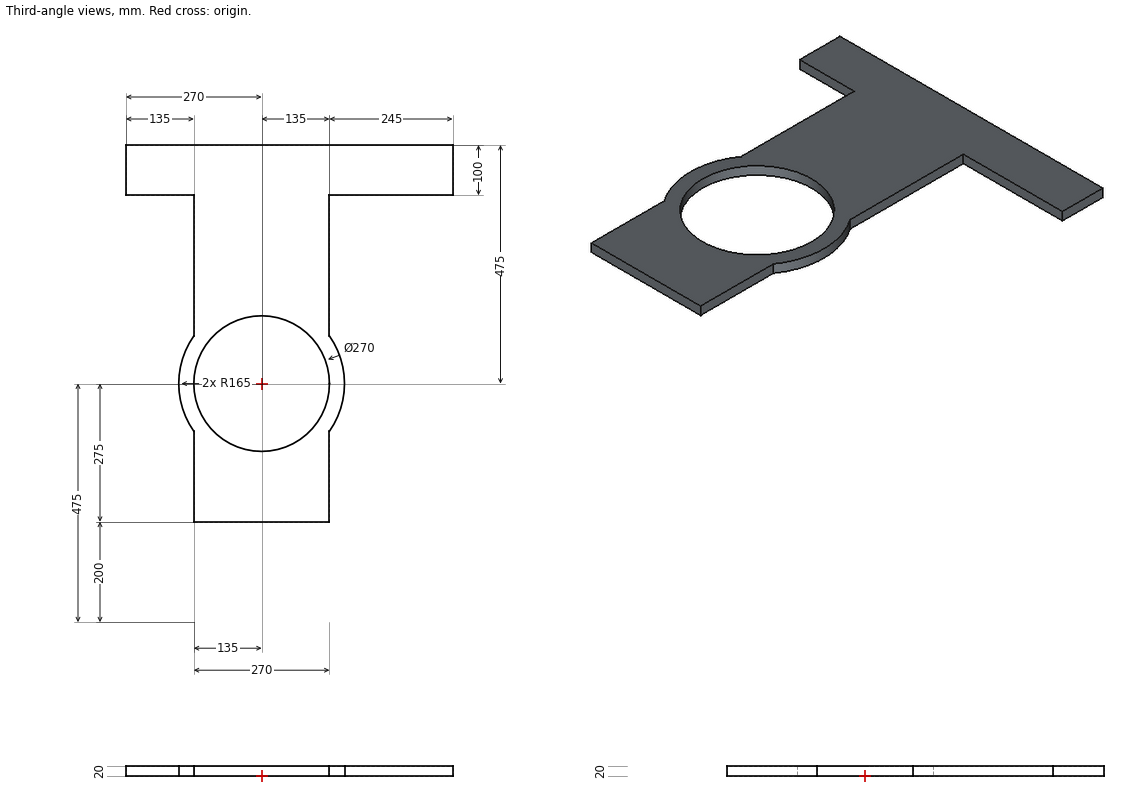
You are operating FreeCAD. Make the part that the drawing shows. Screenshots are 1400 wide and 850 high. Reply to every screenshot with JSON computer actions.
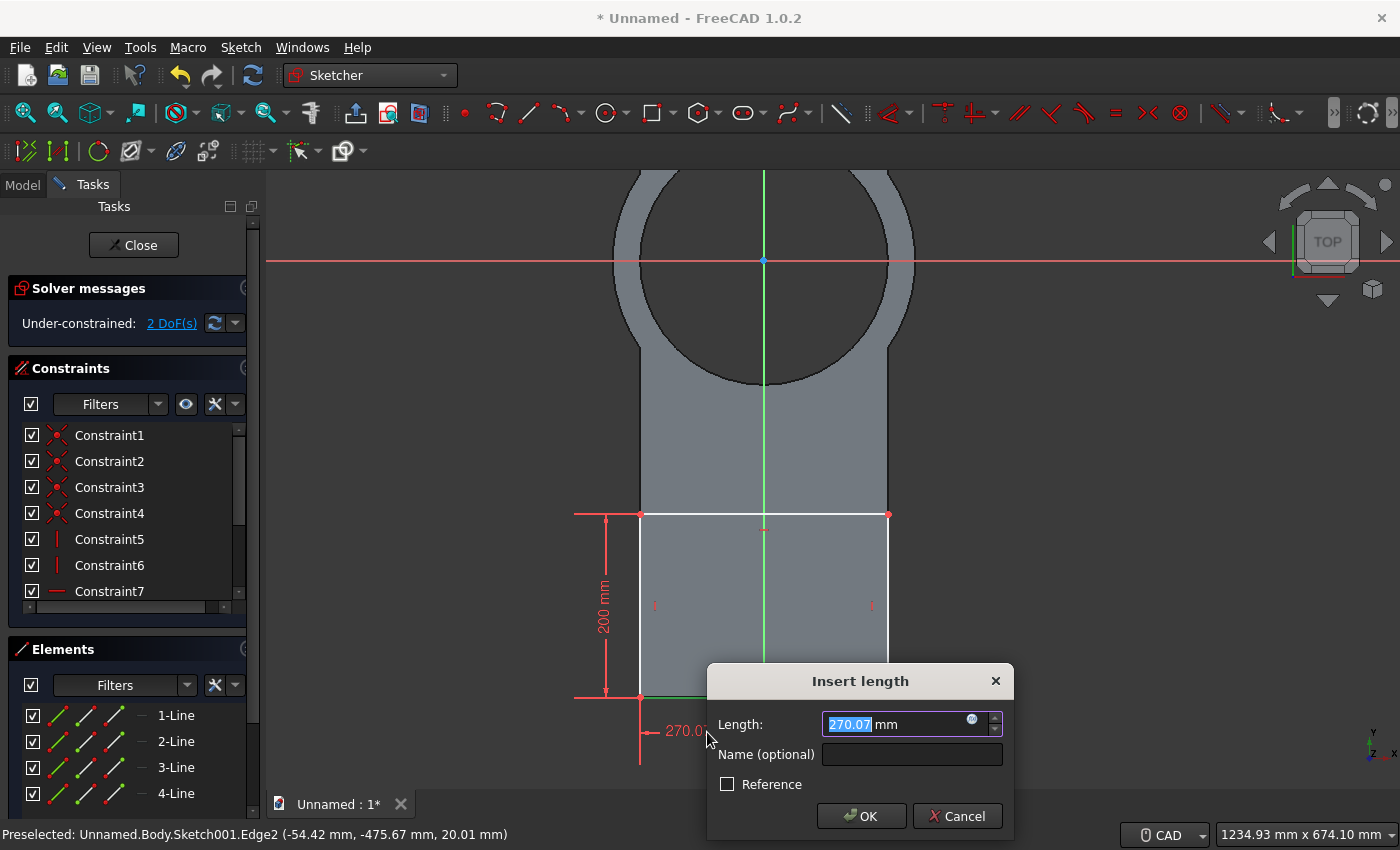
{"action": "type", "text": "270"}
{"action": "key", "text": "Return"}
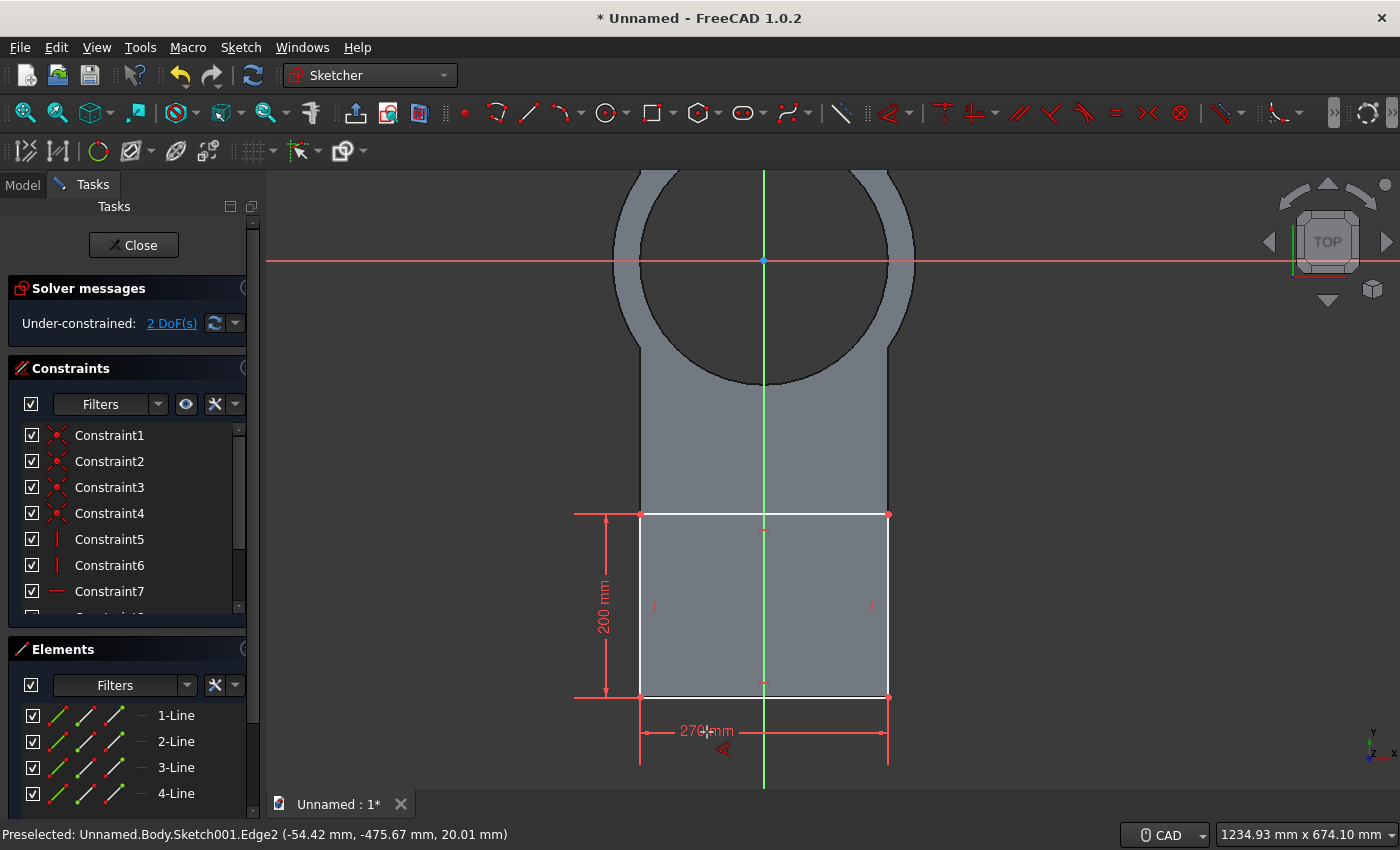
{"action": "left_click", "coordinate": [640, 514]}
{"action": "left_click", "coordinate": [702, 227]}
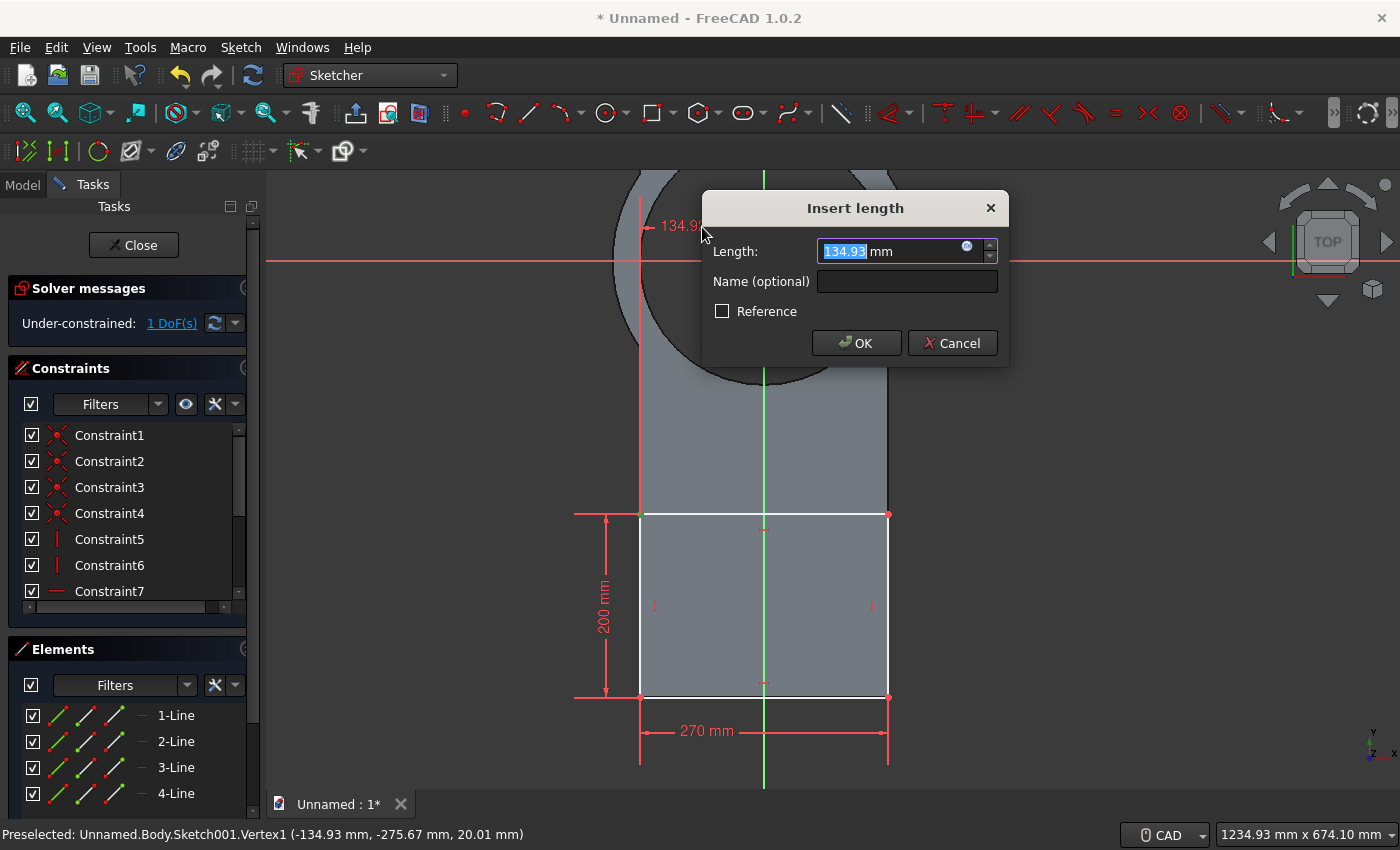
{"action": "type", "text": "135"}
{"action": "key", "text": "Return"}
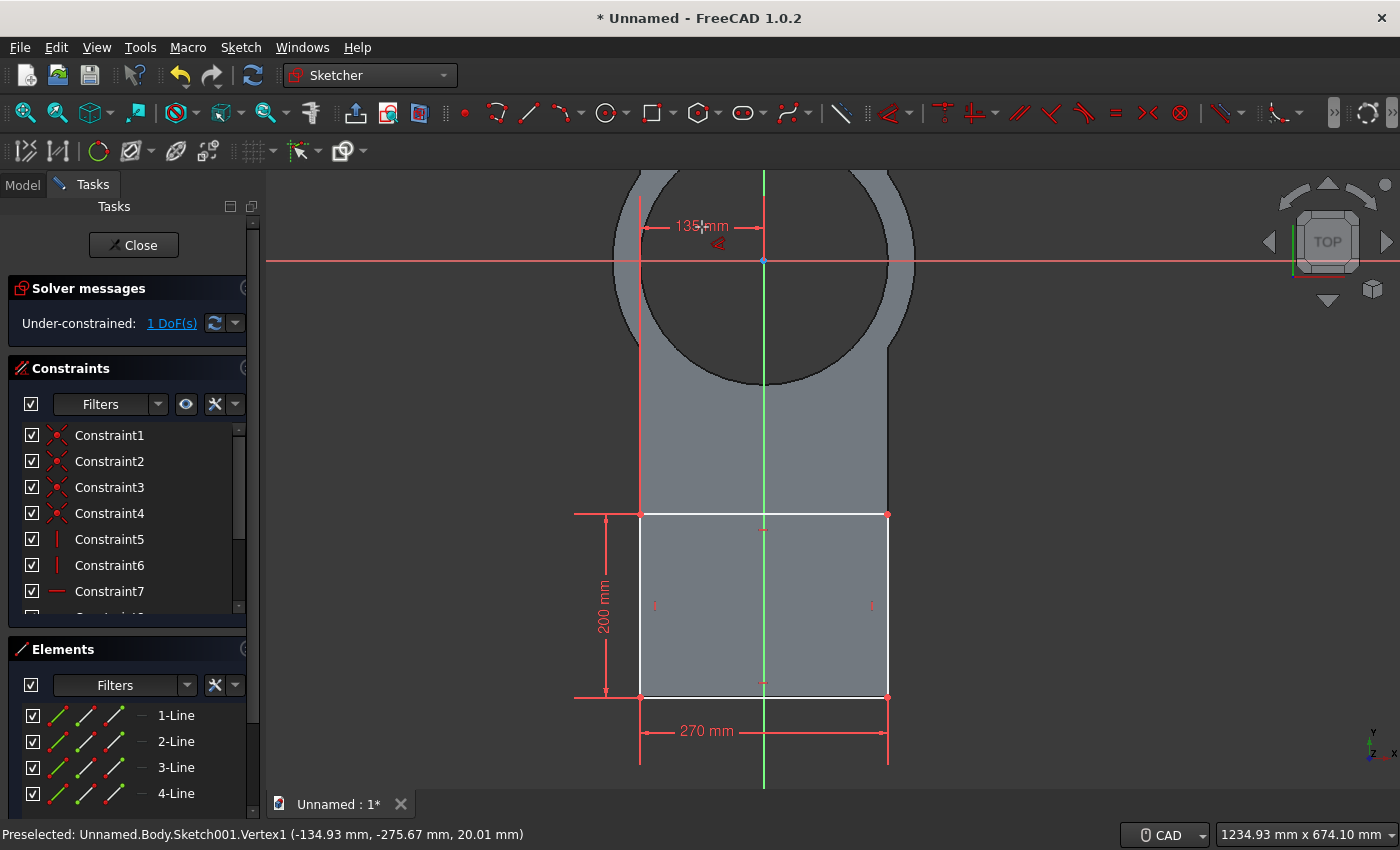
{"action": "left_click", "coordinate": [640, 514]}
{"action": "left_click", "coordinate": [606, 387]}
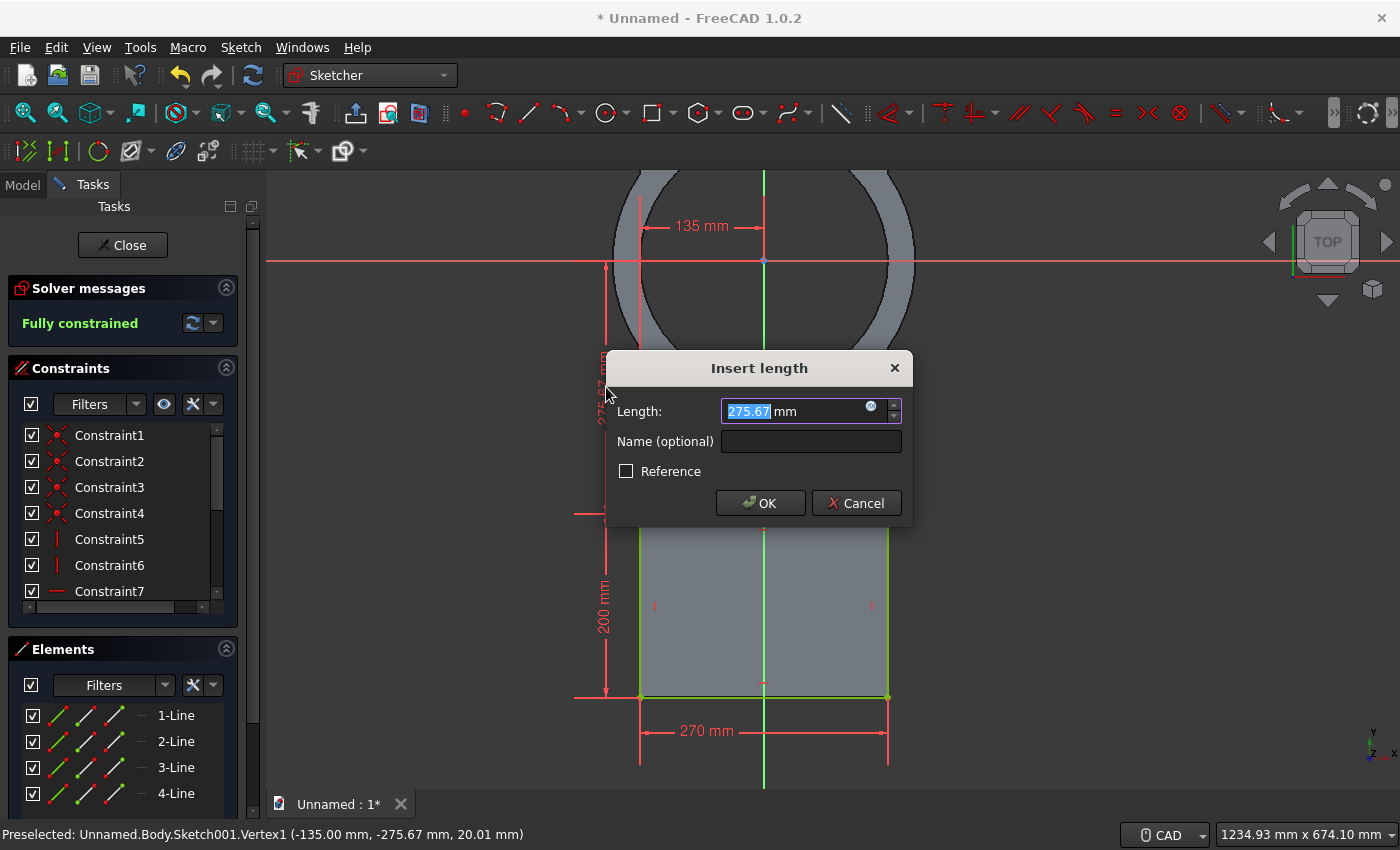
{"action": "type", "text": "275"}
{"action": "key", "text": "Return"}
{"action": "key", "text": "Escape"}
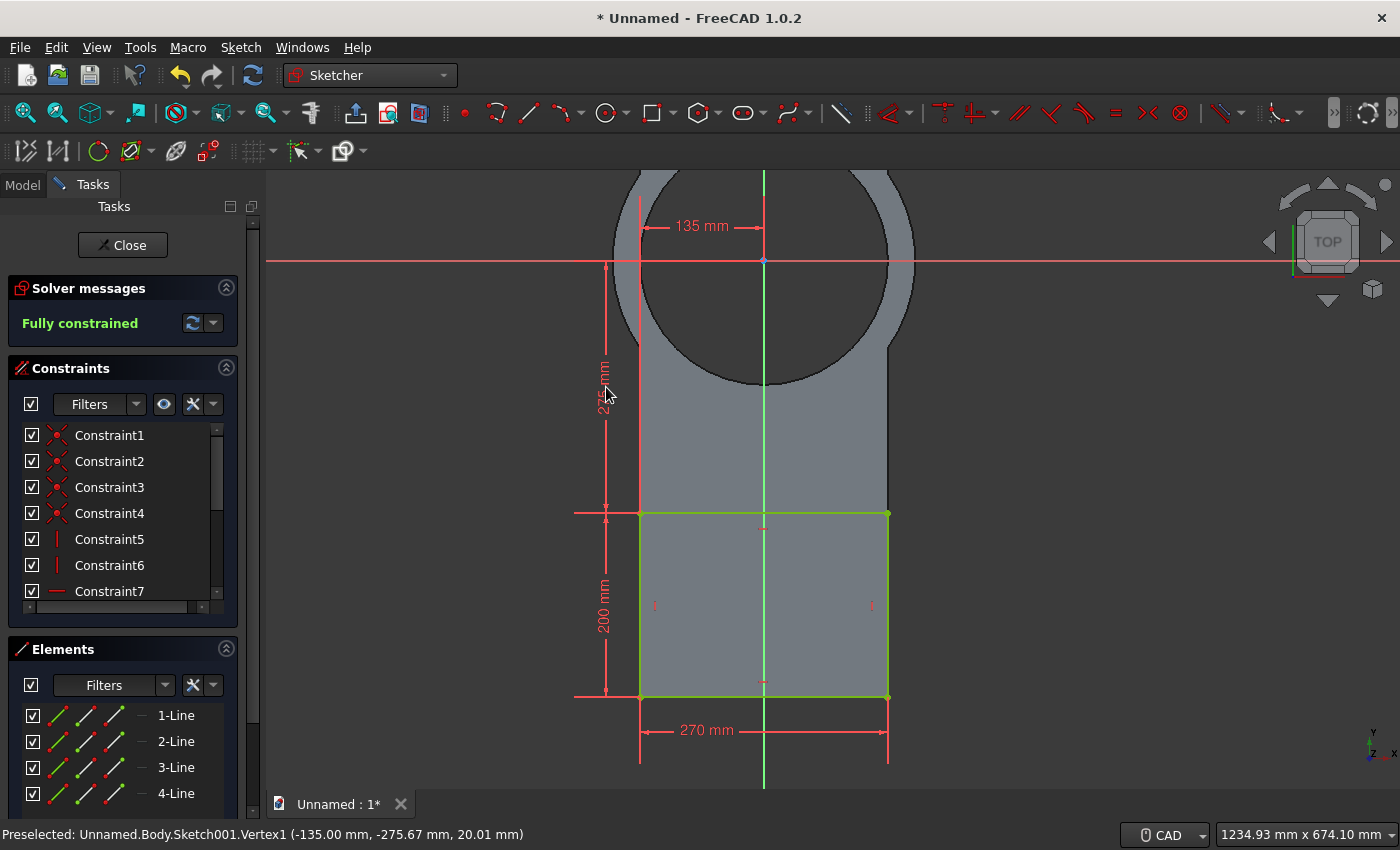
{"action": "left_click", "coordinate": [123, 245]}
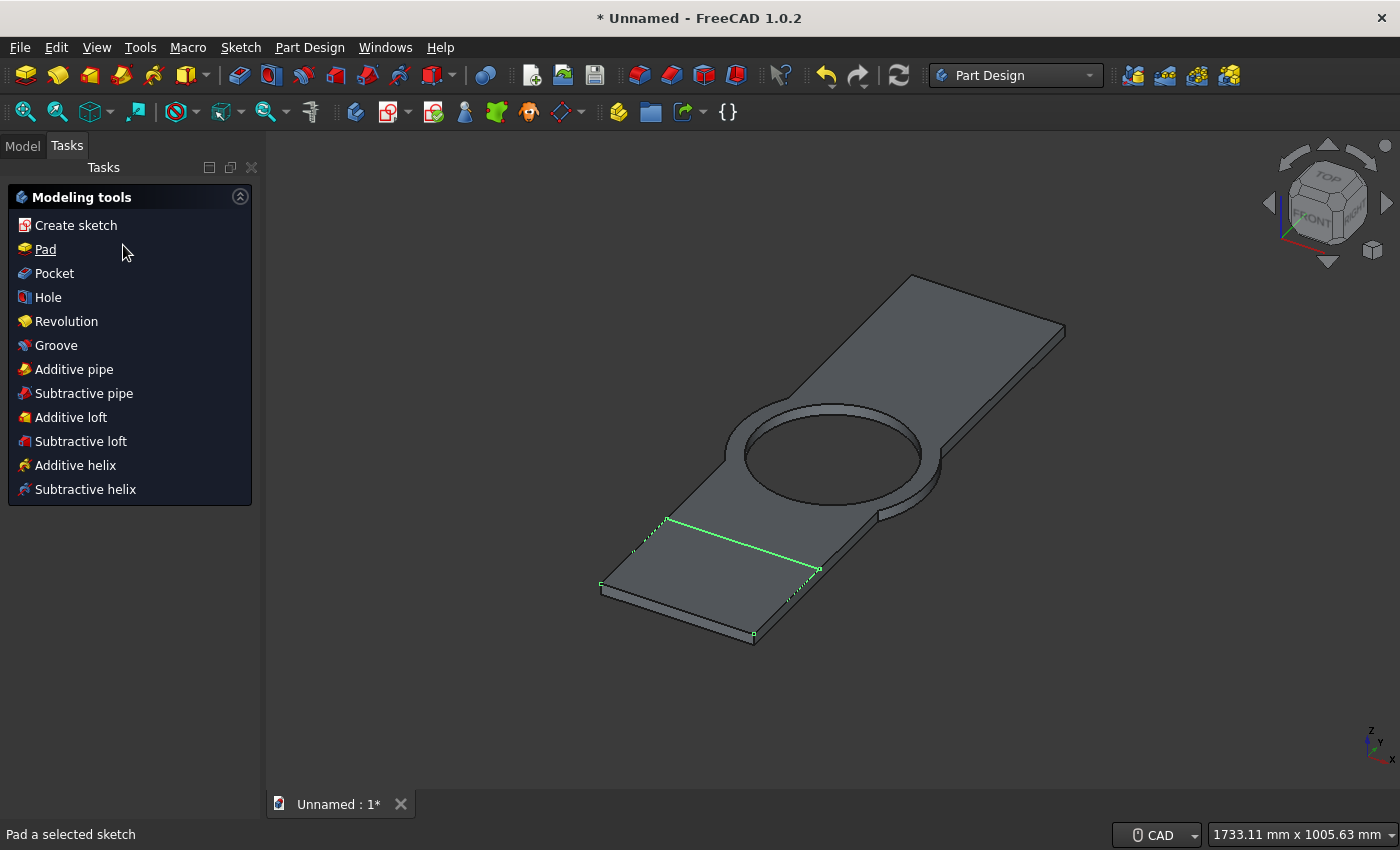
{"action": "left_click", "coordinate": [240, 76]}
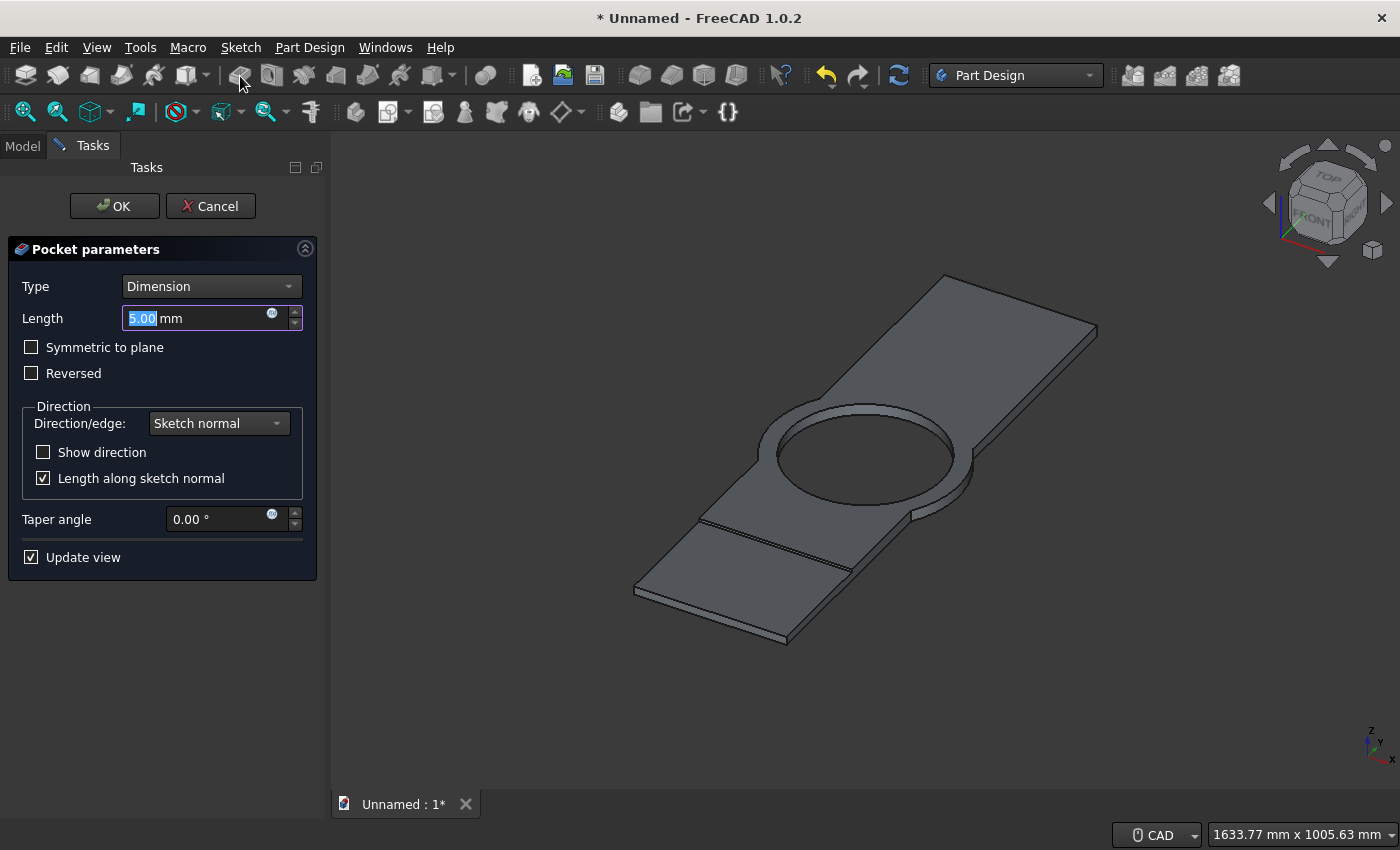
{"action": "type", "text": "20"}
{"action": "key", "text": "Tab"}